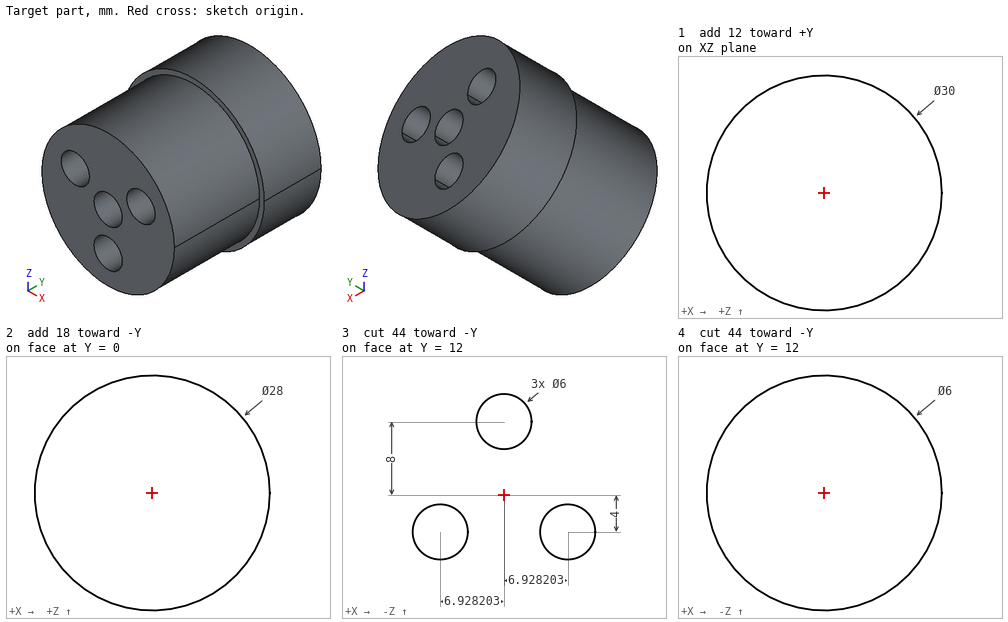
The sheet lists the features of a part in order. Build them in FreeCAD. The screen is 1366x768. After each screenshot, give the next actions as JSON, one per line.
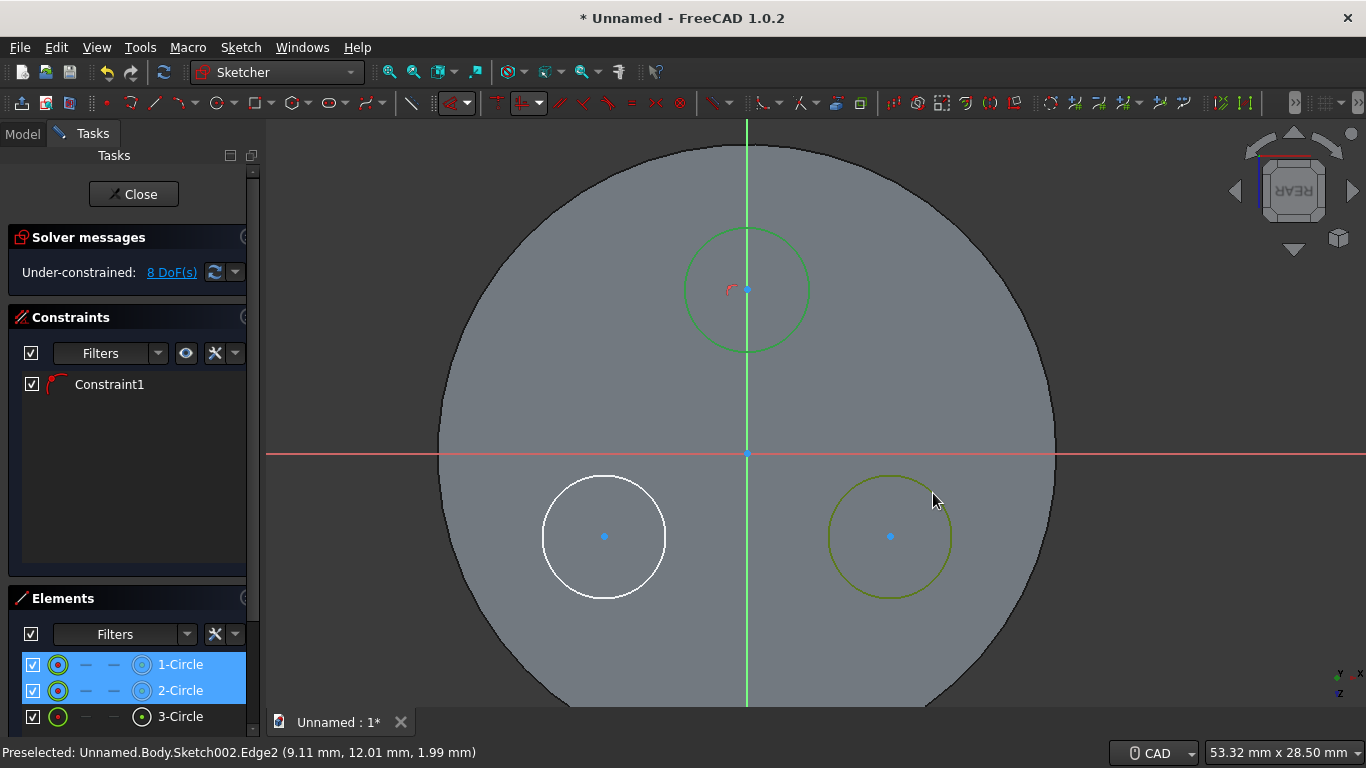
{"action": "left_click", "coordinate": [647, 493]}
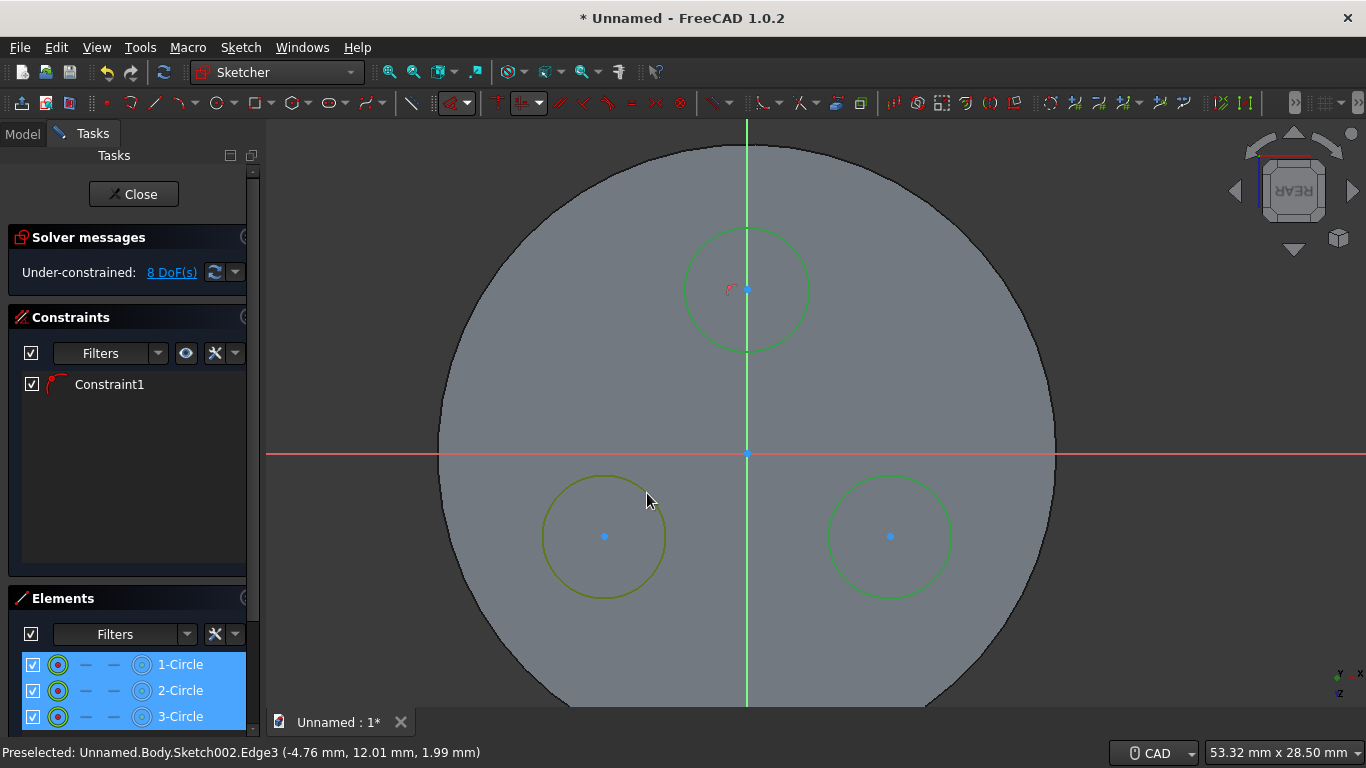
{"action": "left_click", "coordinate": [632, 104]}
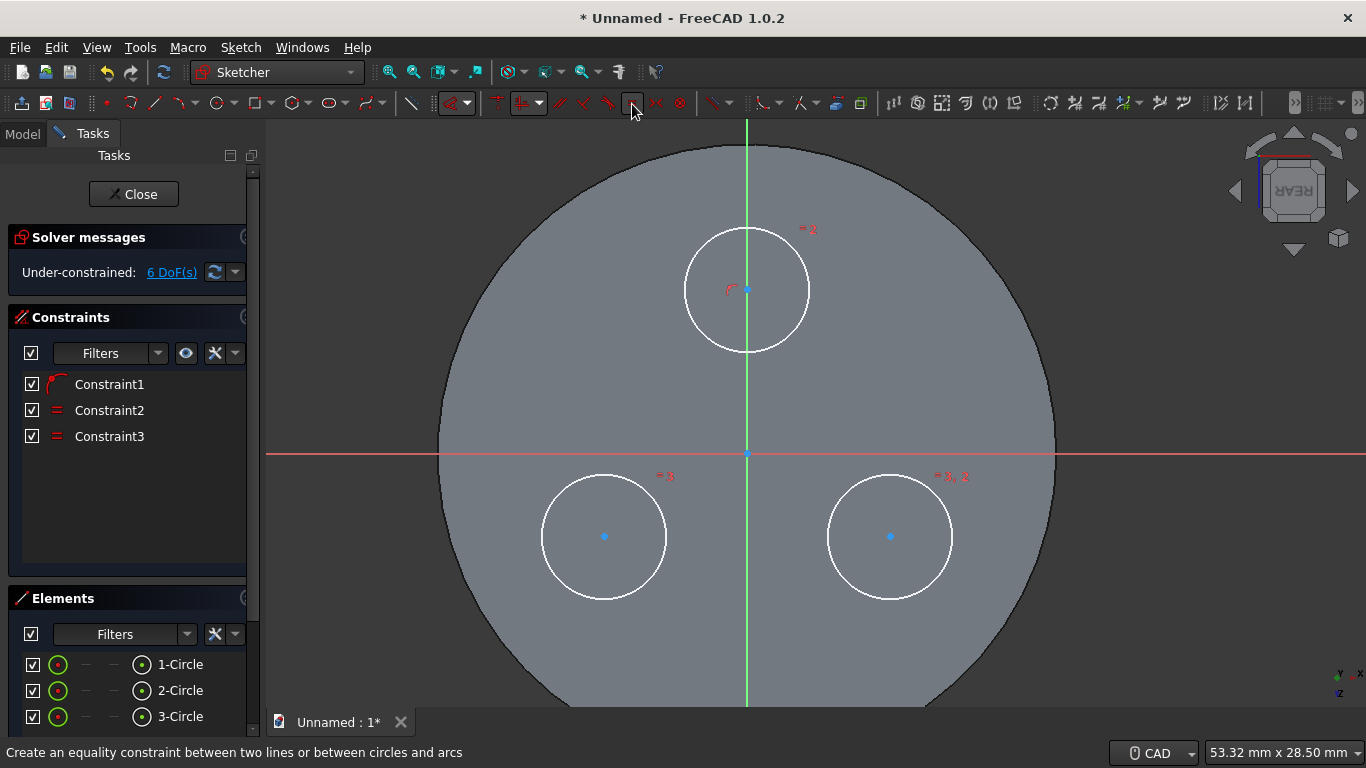
{"action": "left_click", "coordinate": [890, 537]}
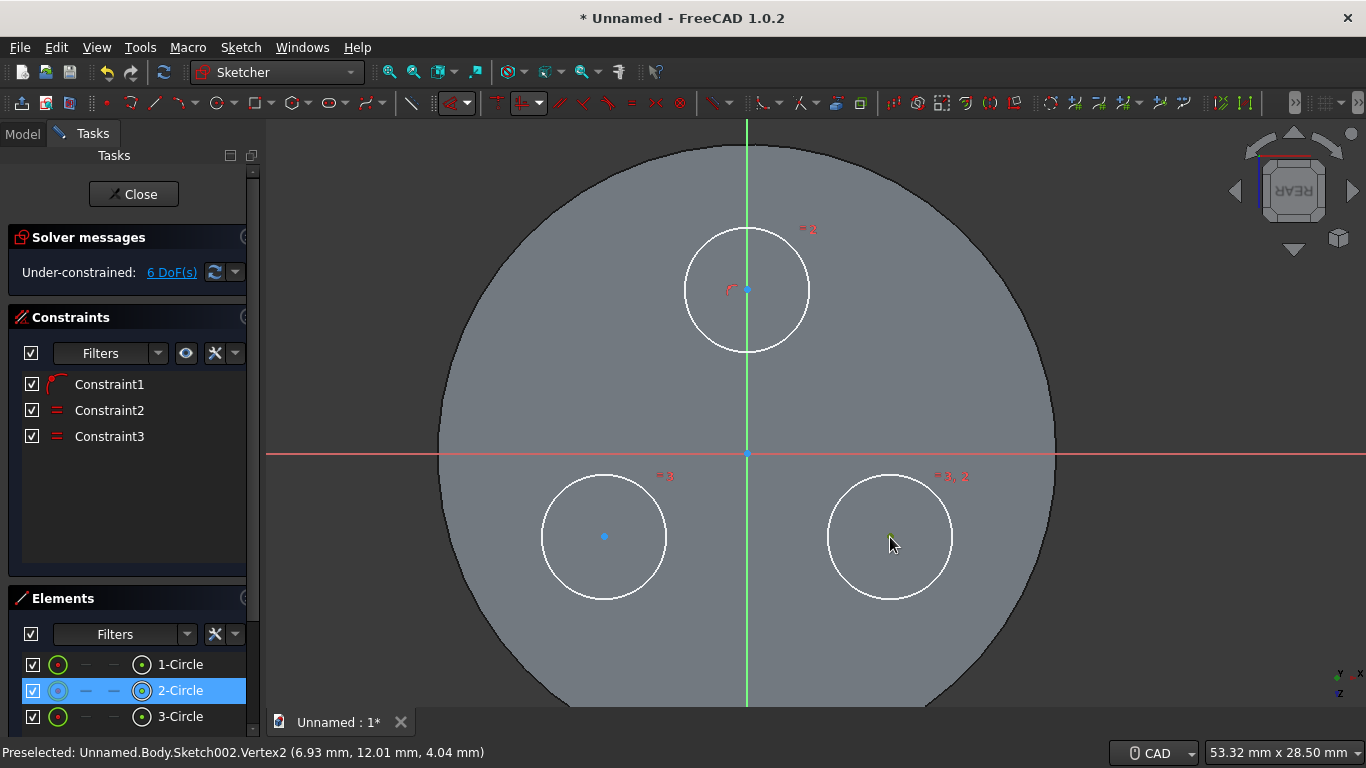
{"action": "left_click", "coordinate": [604, 537]}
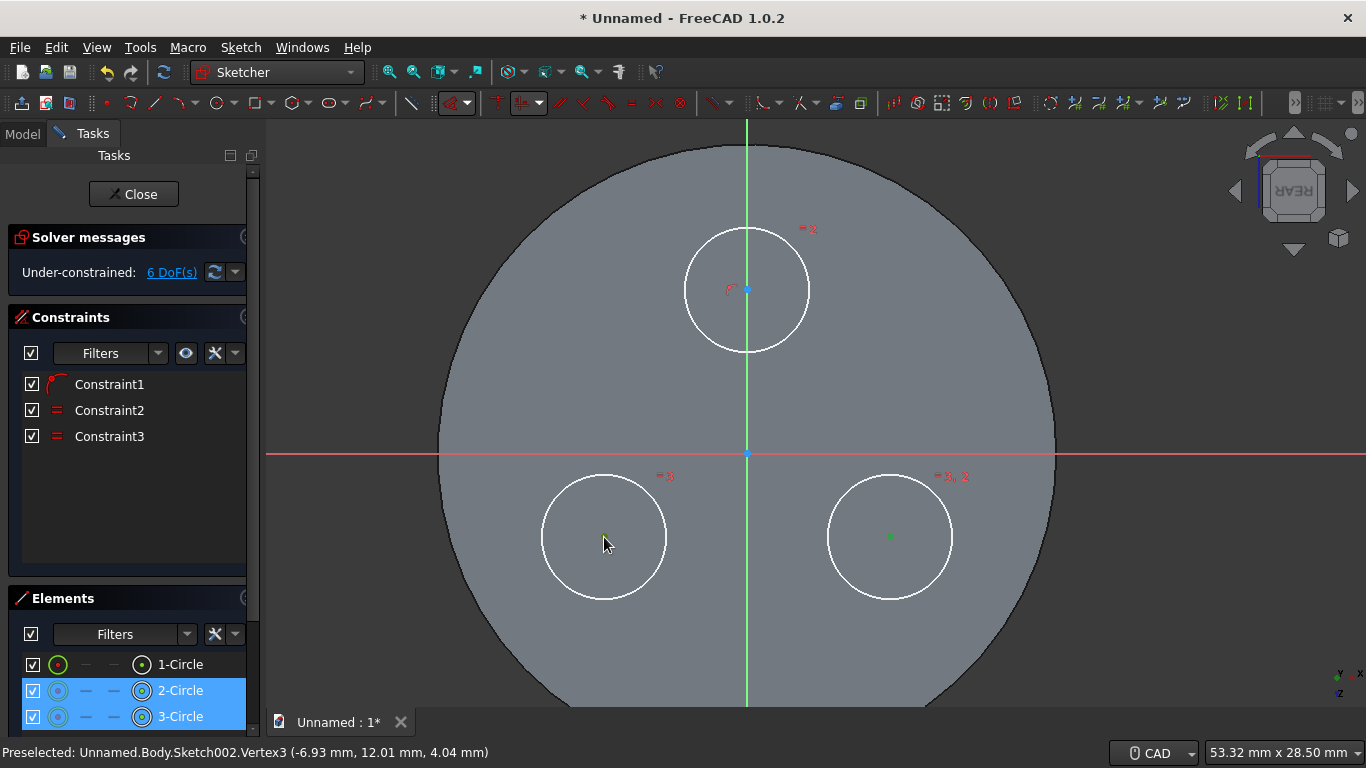
{"action": "key", "text": "h"}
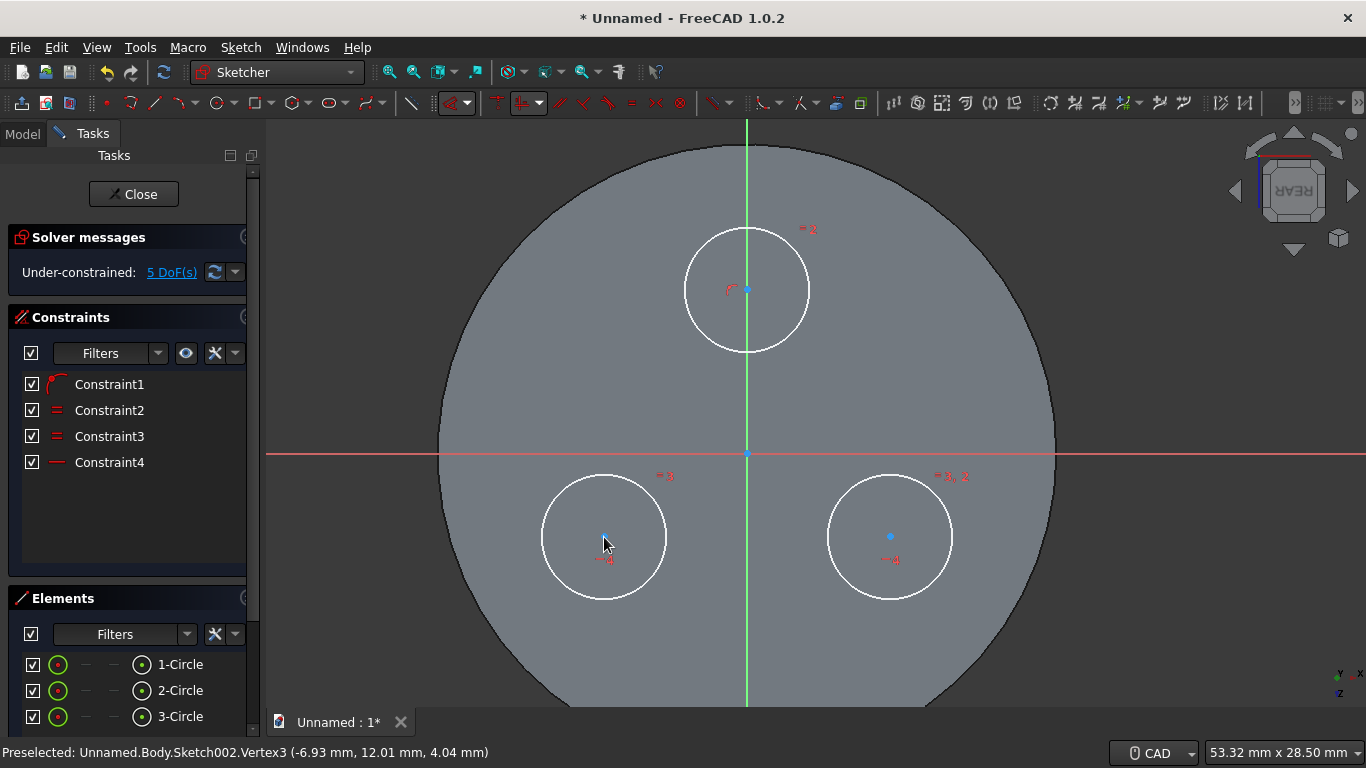
{"action": "left_click", "coordinate": [791, 246]}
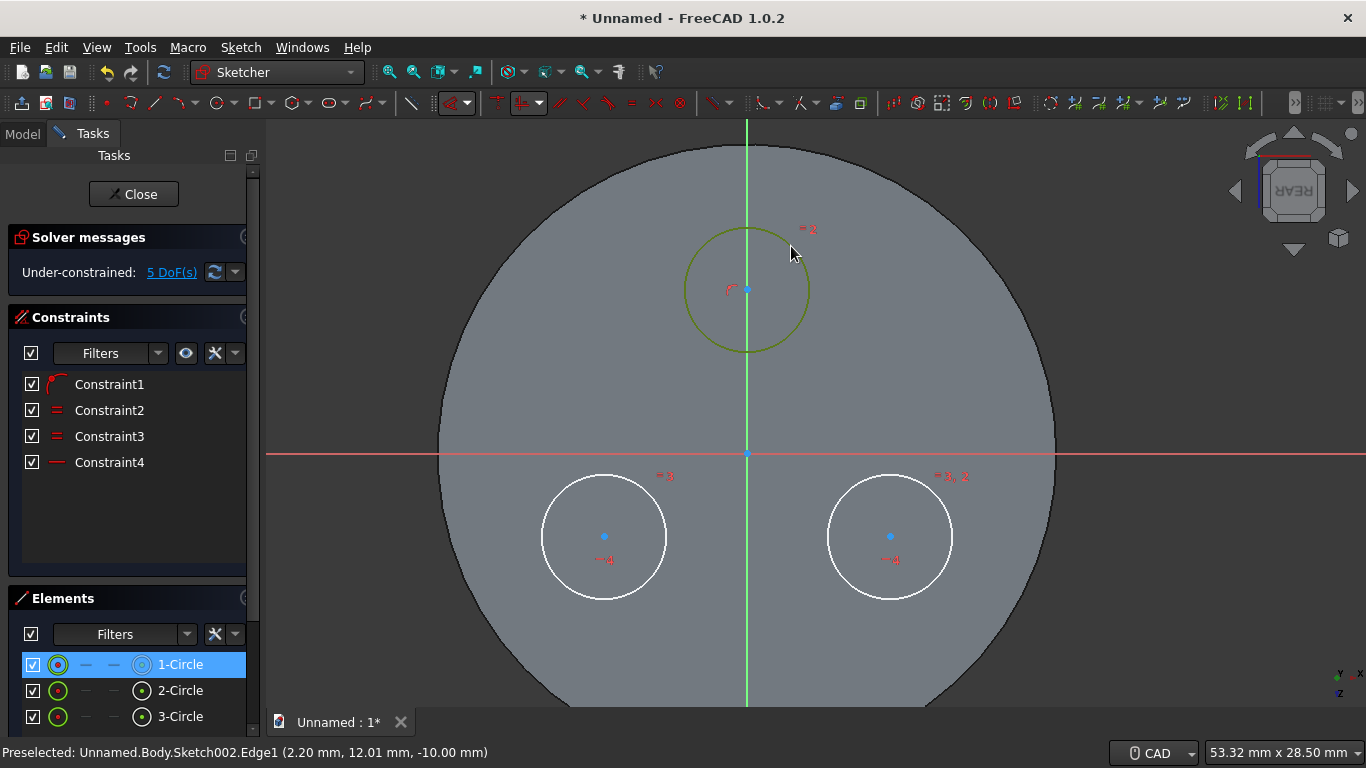
{"action": "left_click", "coordinate": [470, 104]}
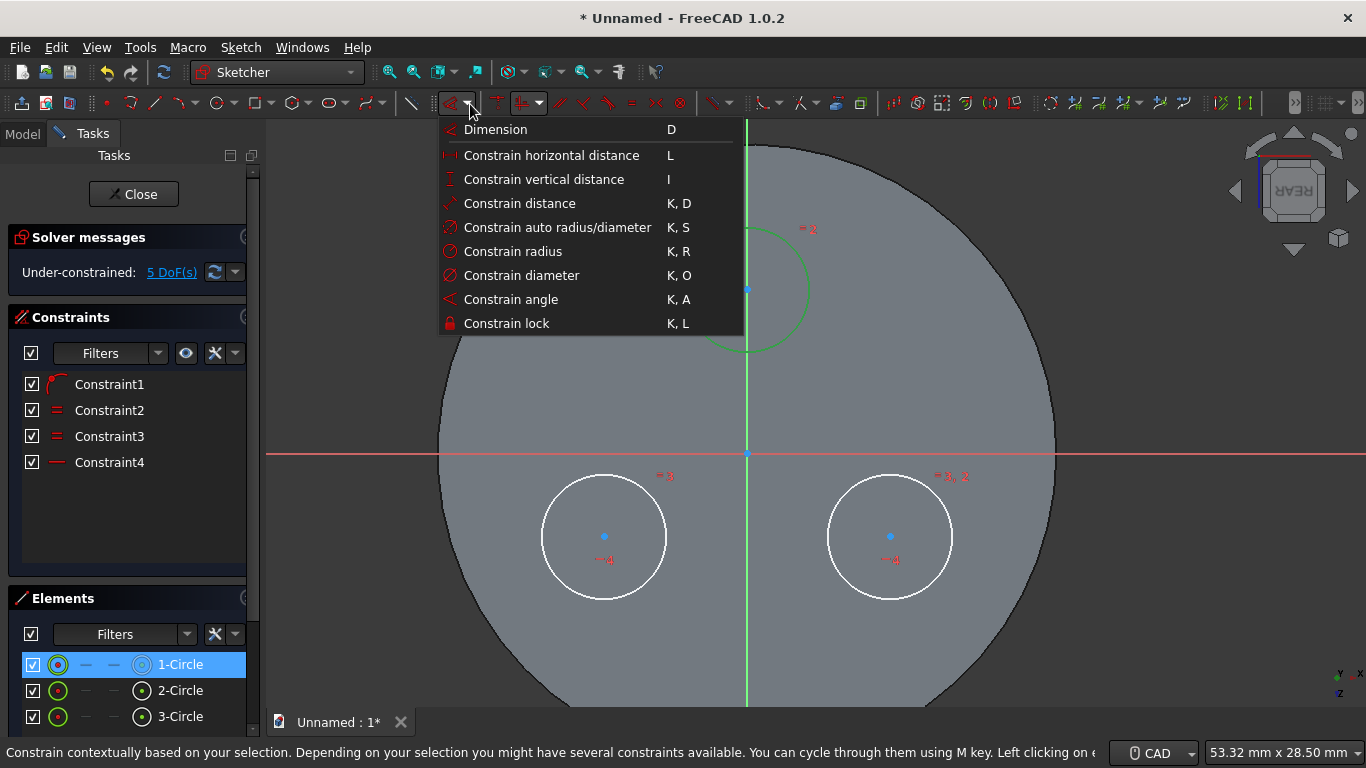
{"action": "left_click", "coordinate": [591, 275]}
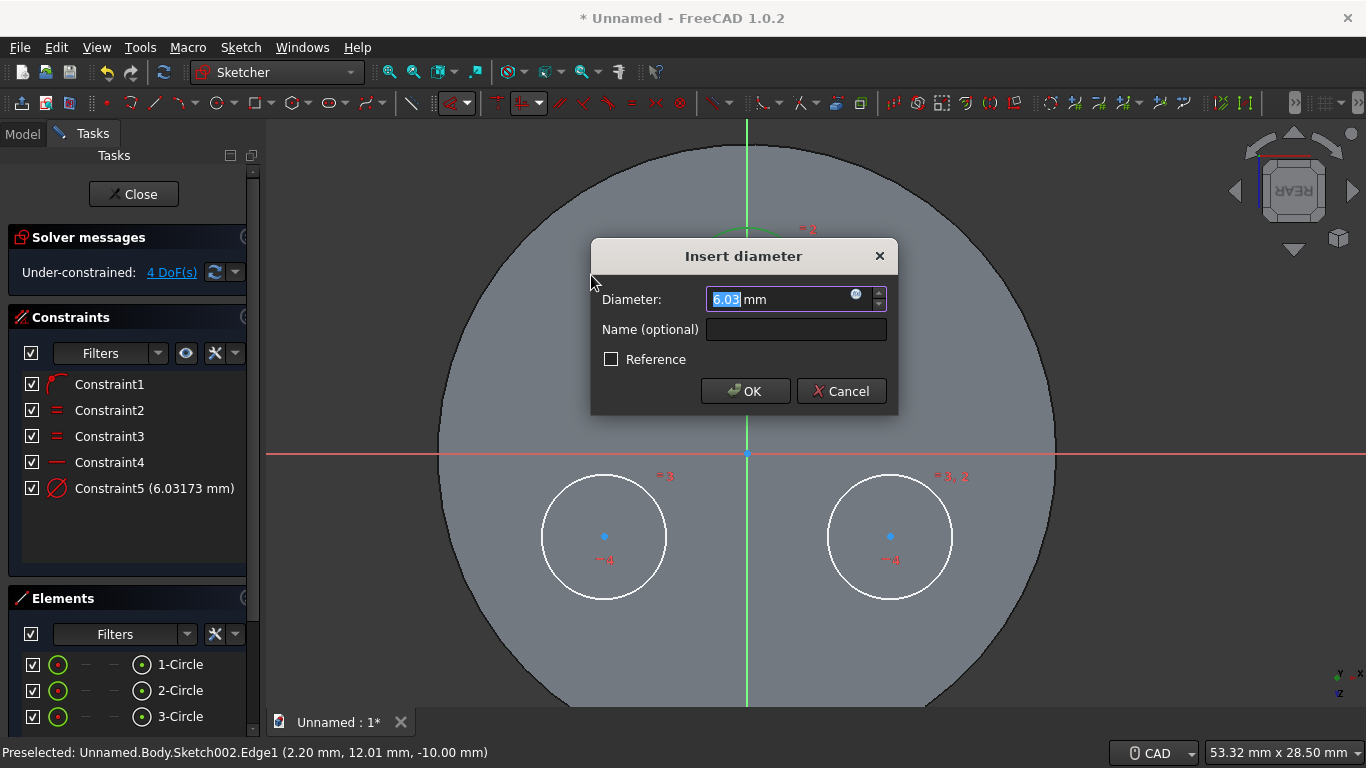
{"action": "type", "text": "6"}
{"action": "key", "text": "Return"}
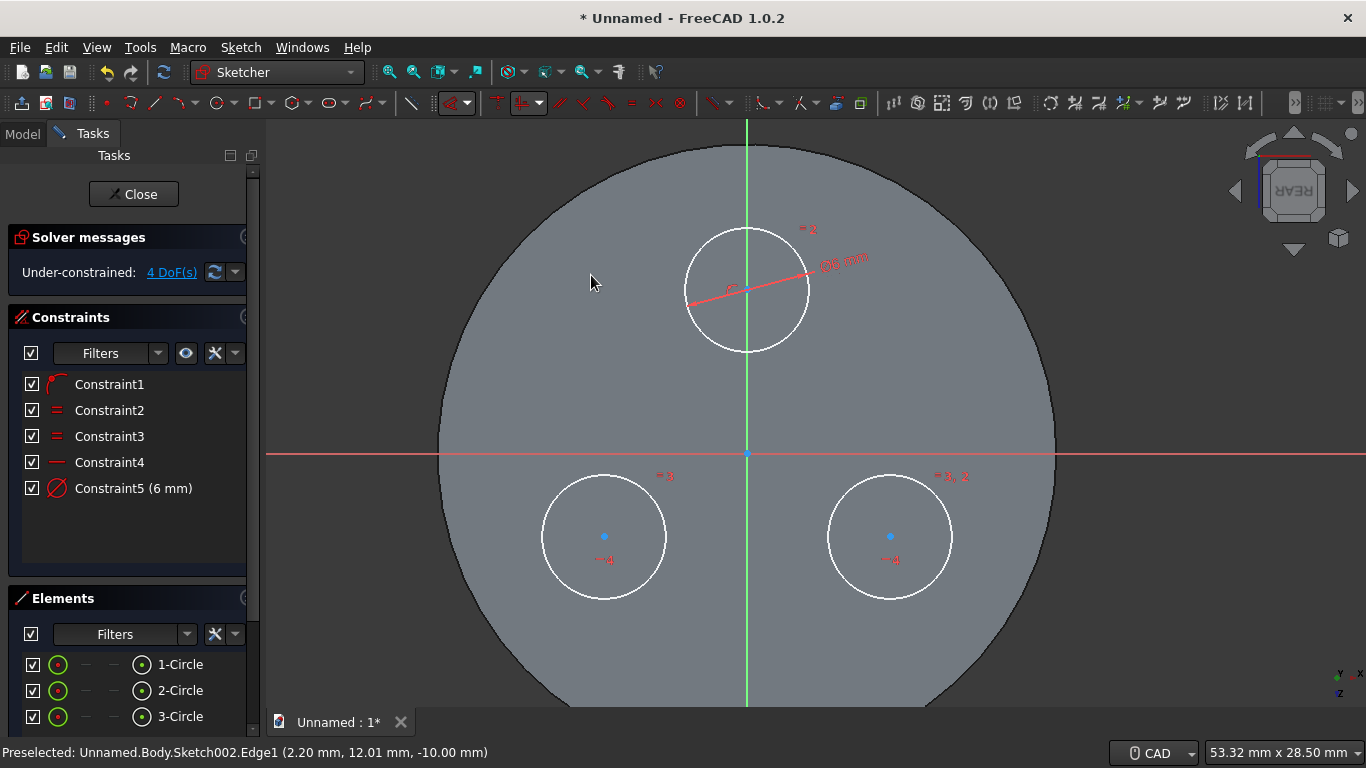
{"action": "left_click", "coordinate": [747, 290]}